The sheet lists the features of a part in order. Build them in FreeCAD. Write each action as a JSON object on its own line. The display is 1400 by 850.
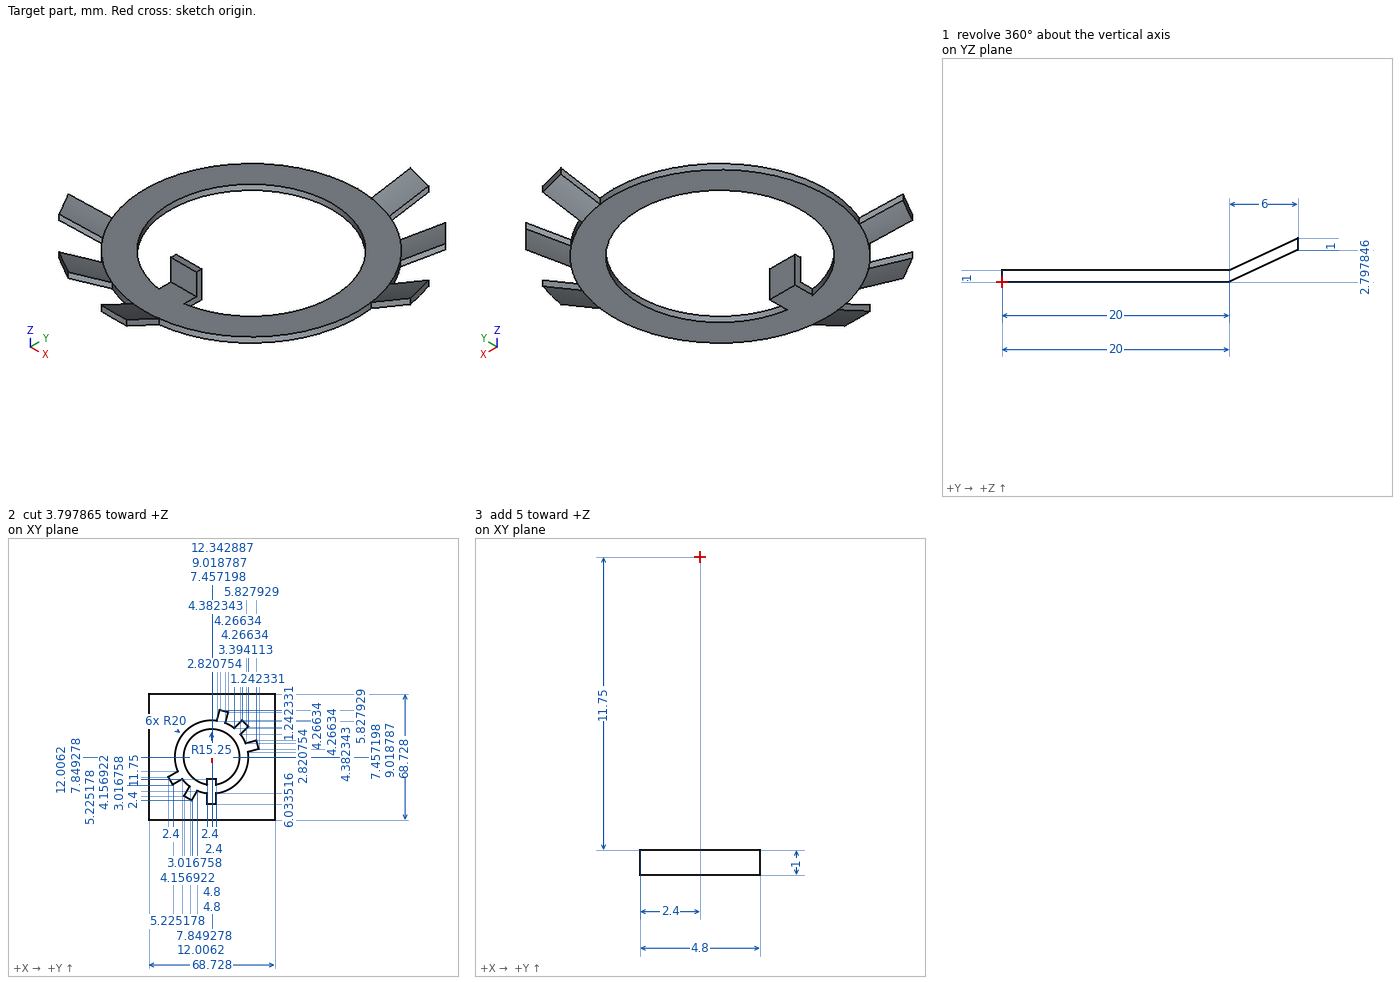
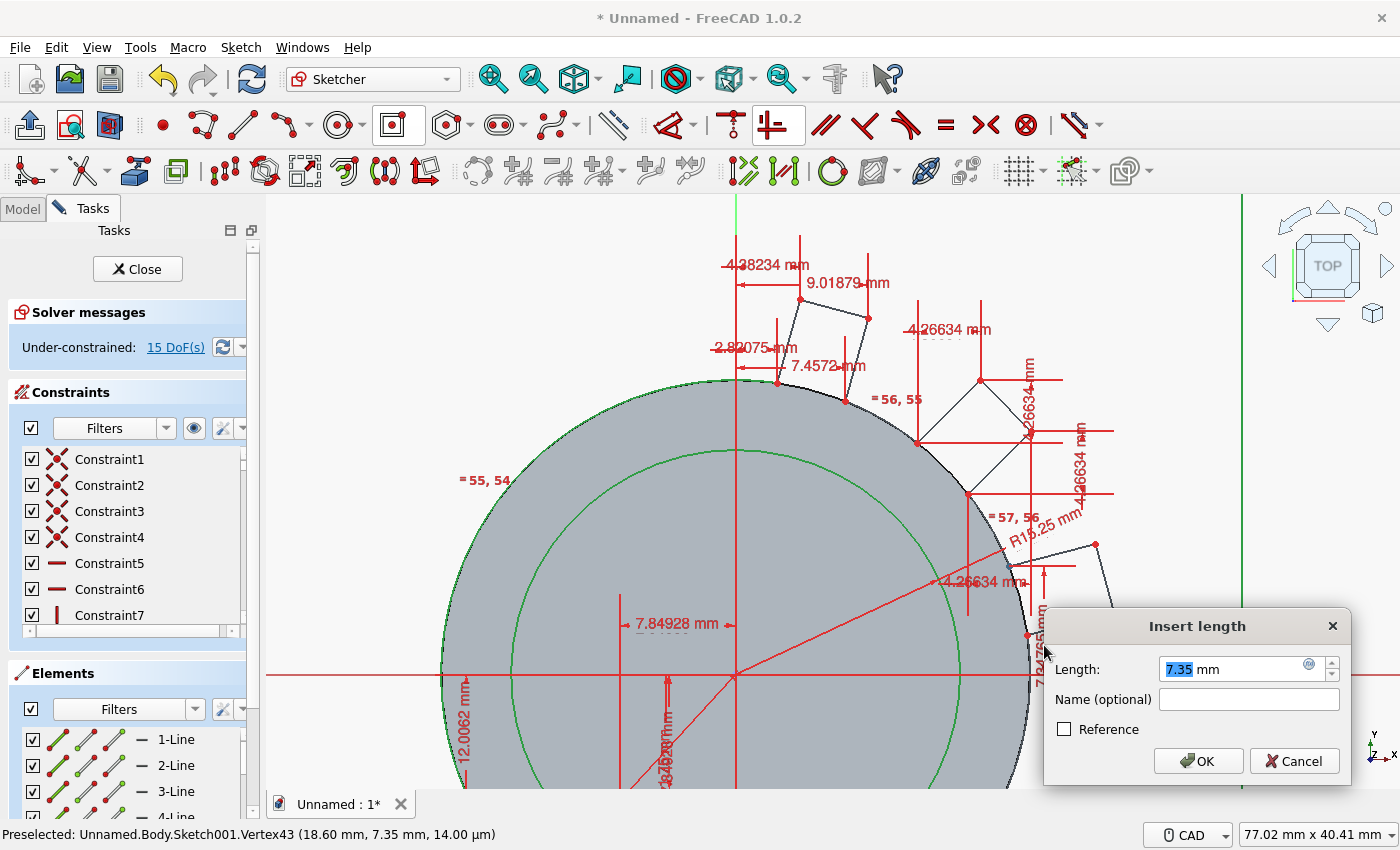
{"action": "type", "text": "7.457198"}
{"action": "key", "text": "Return"}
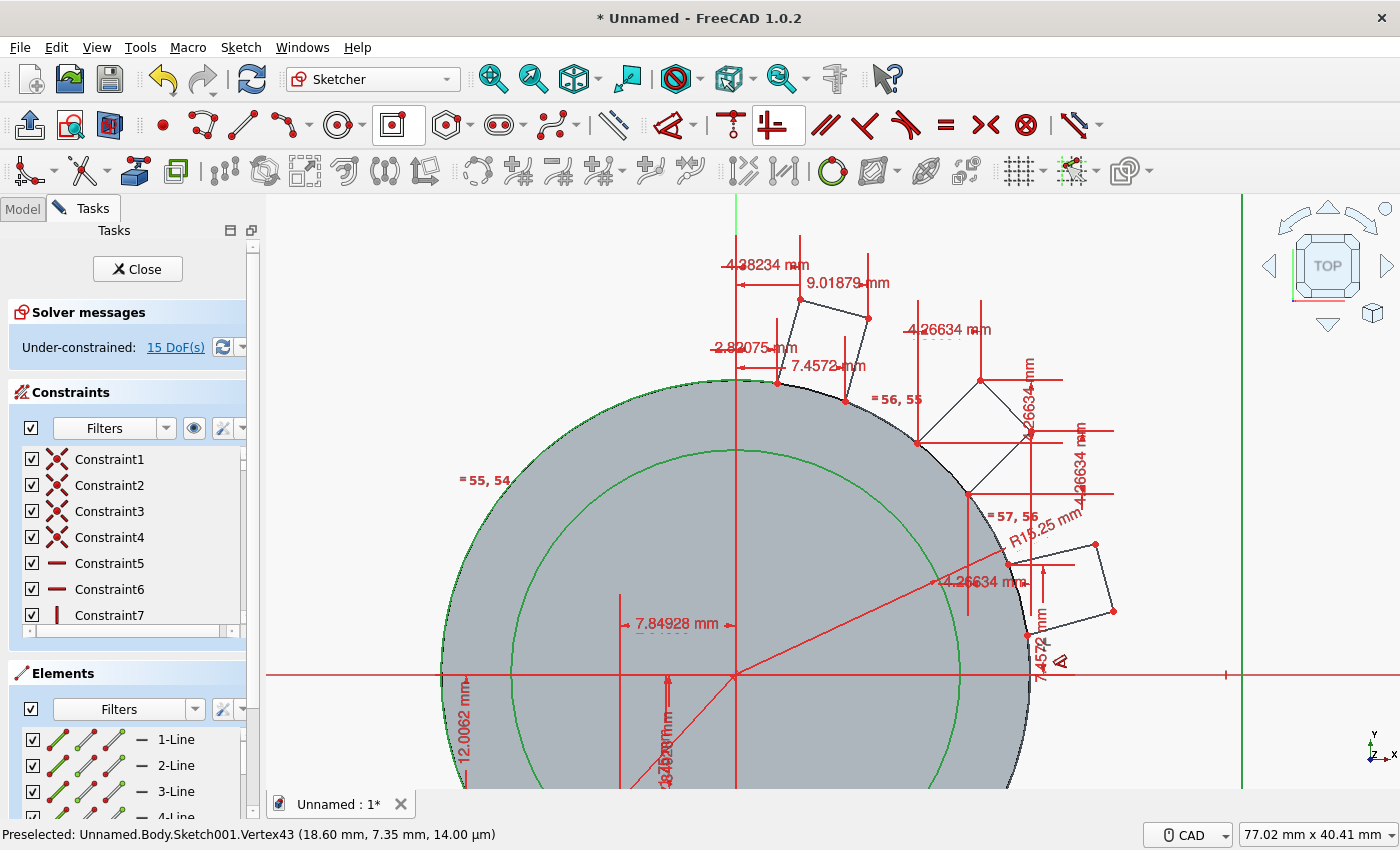
{"action": "left_click", "coordinate": [1096, 544]}
{"action": "left_click", "coordinate": [1130, 609]}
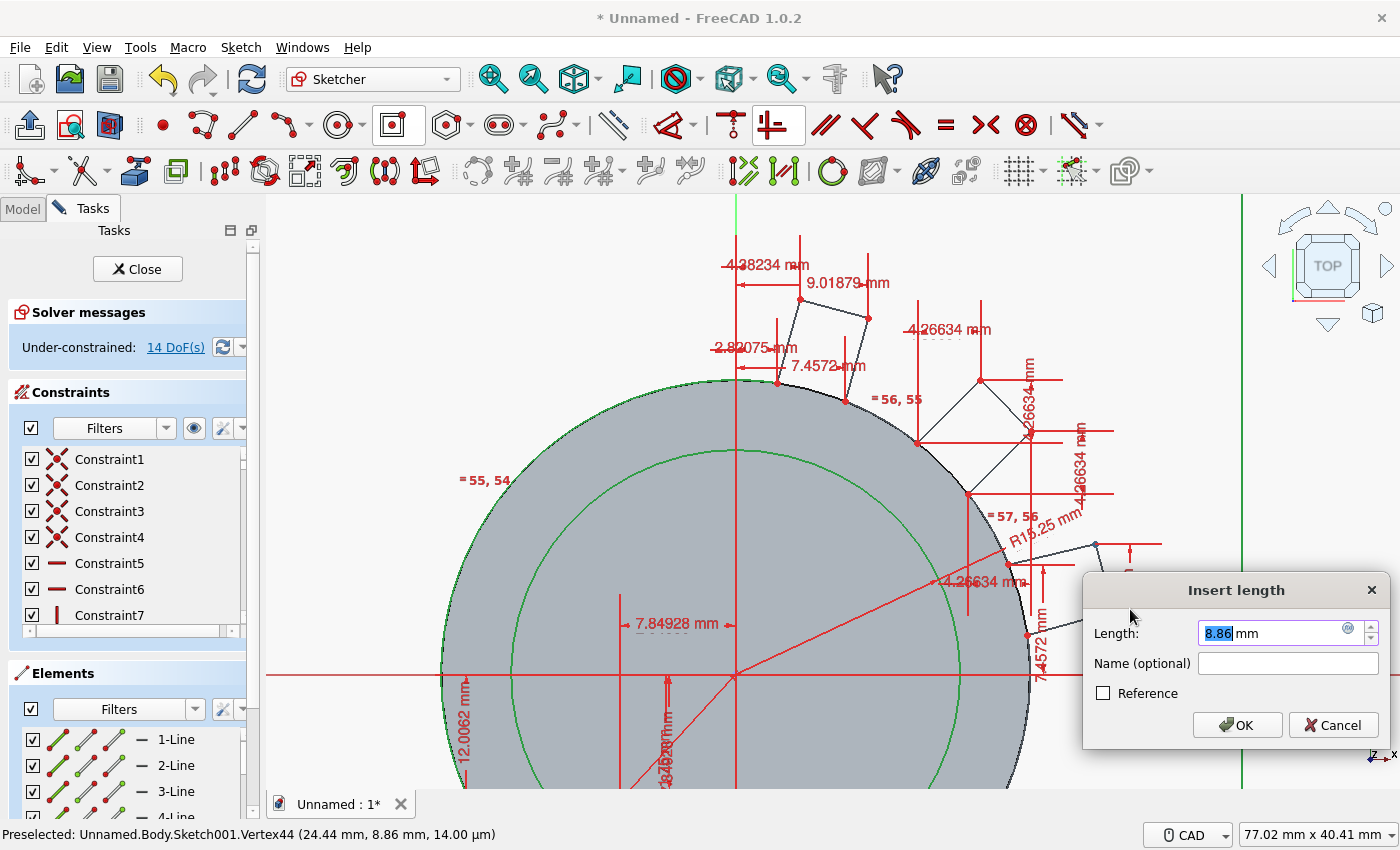
{"action": "type", "text": "9.018787"}
{"action": "key", "text": "Return"}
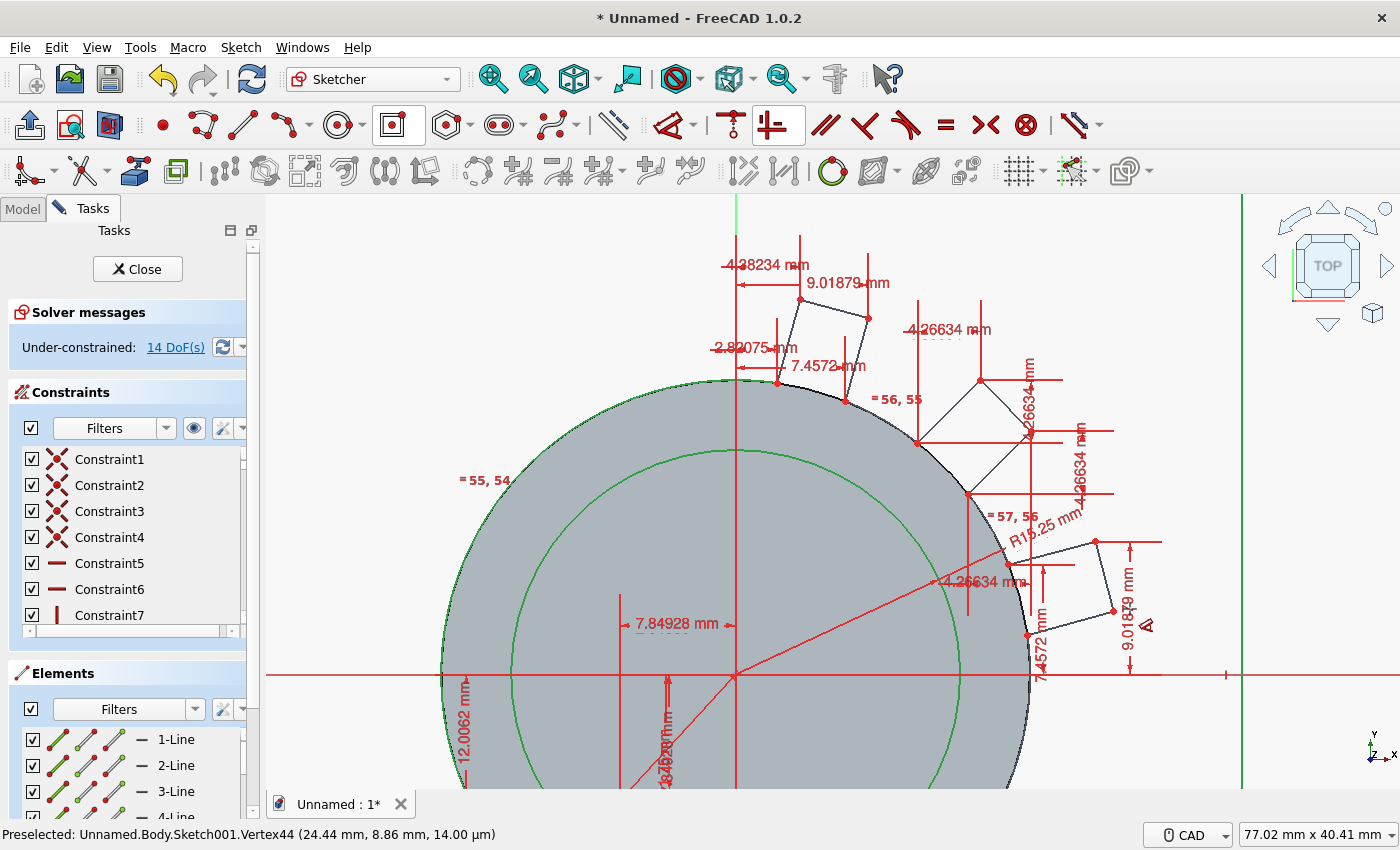
{"action": "left_click", "coordinate": [1114, 611]}
{"action": "left_click", "coordinate": [1148, 643]}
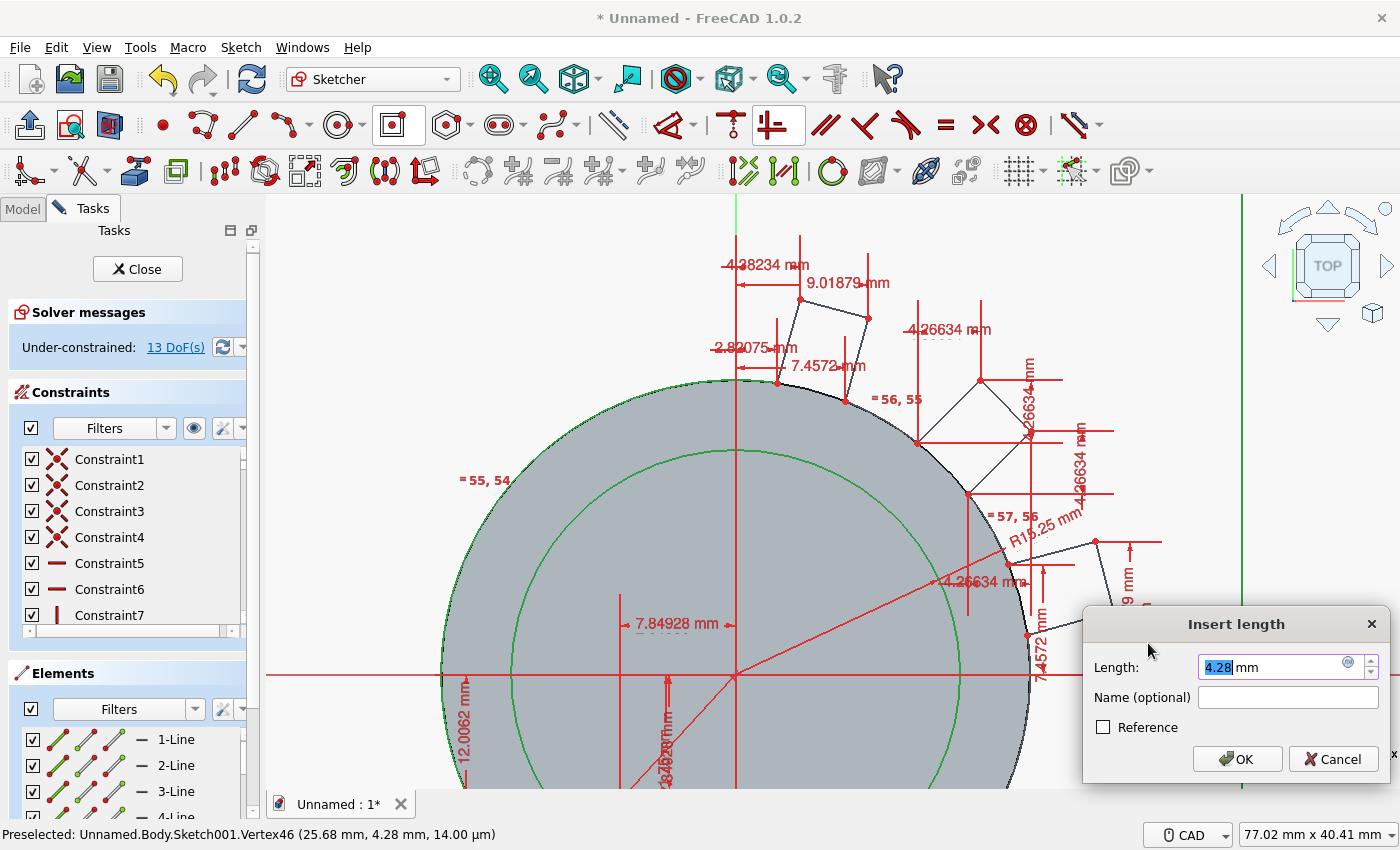
{"action": "type", "text": "4.382343"}
{"action": "key", "text": "Return"}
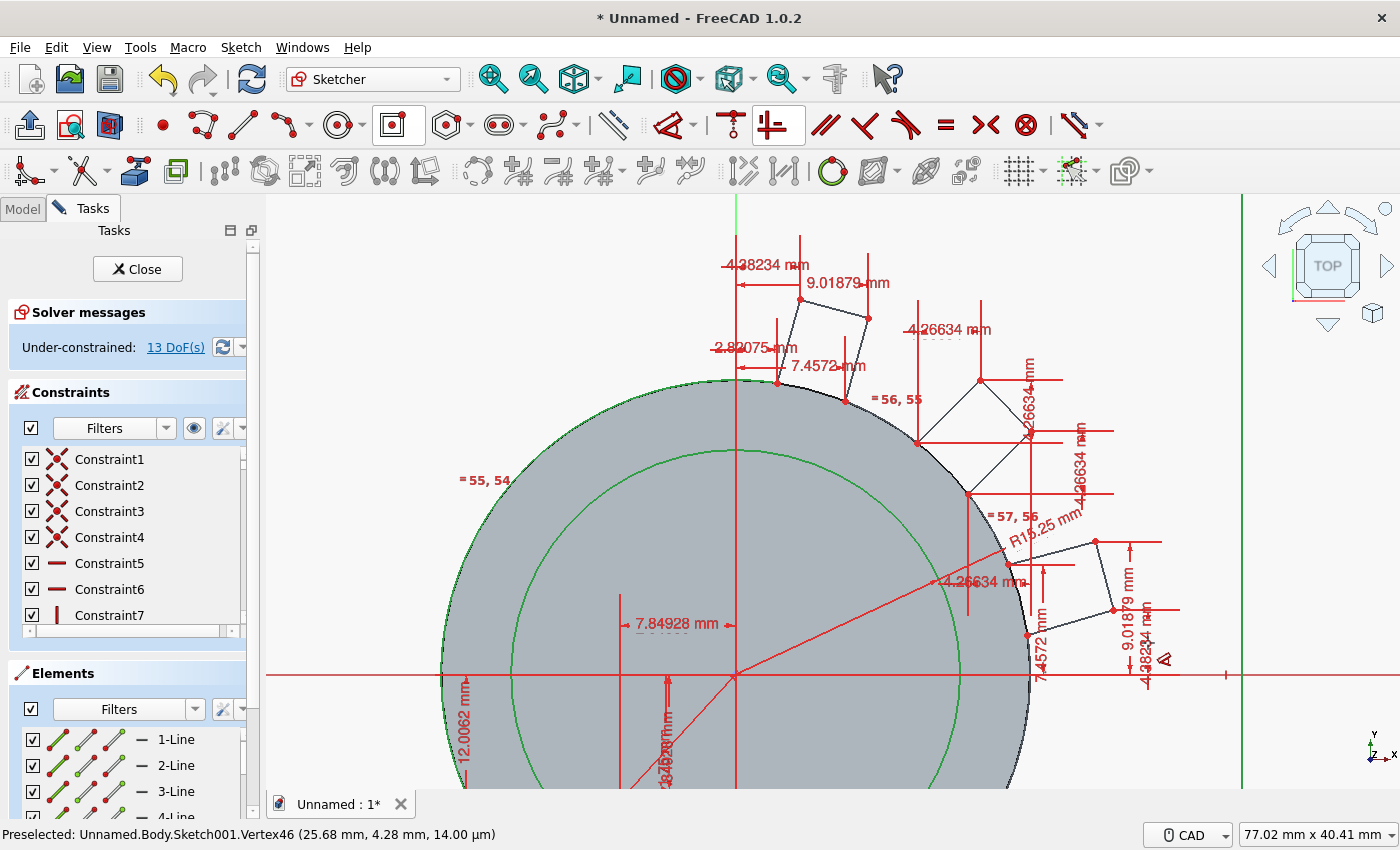
{"action": "left_click", "coordinate": [1027, 635]}
{"action": "left_click", "coordinate": [702, 655]}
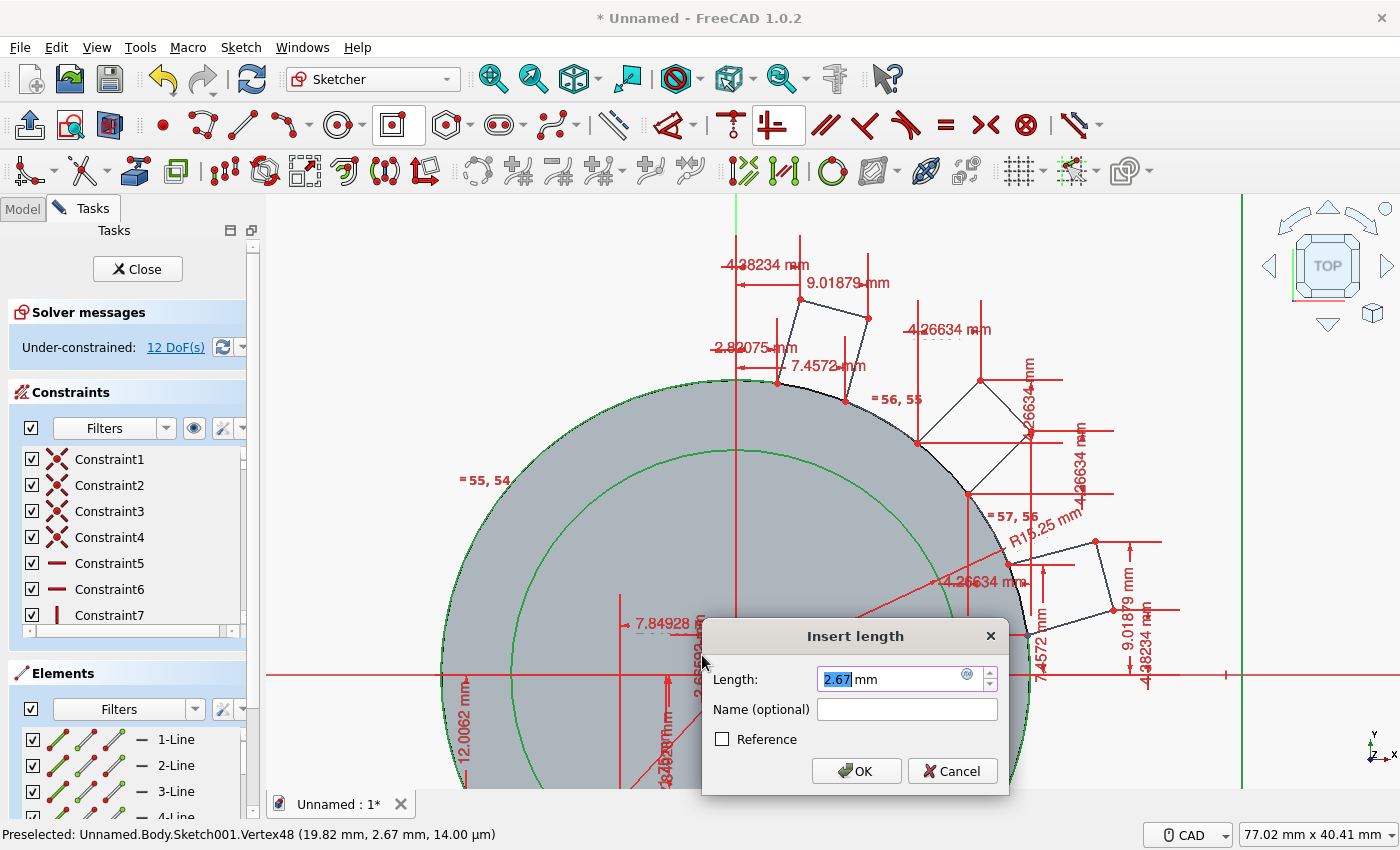
{"action": "type", "text": "2.820754"}
{"action": "key", "text": "Return"}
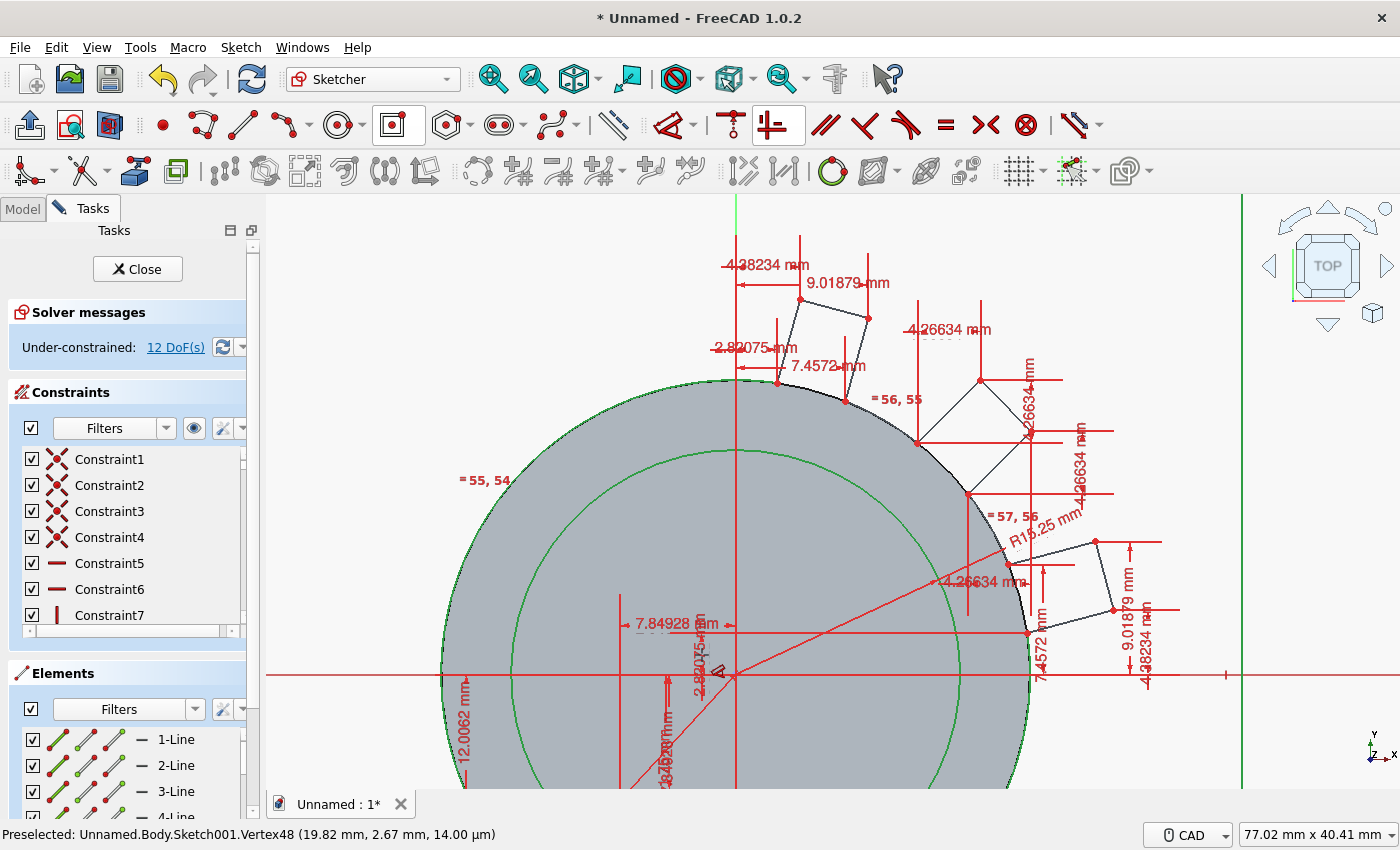
{"action": "scroll", "coordinate": [781, 385], "scroll_direction": "down", "scroll_amount": 5}